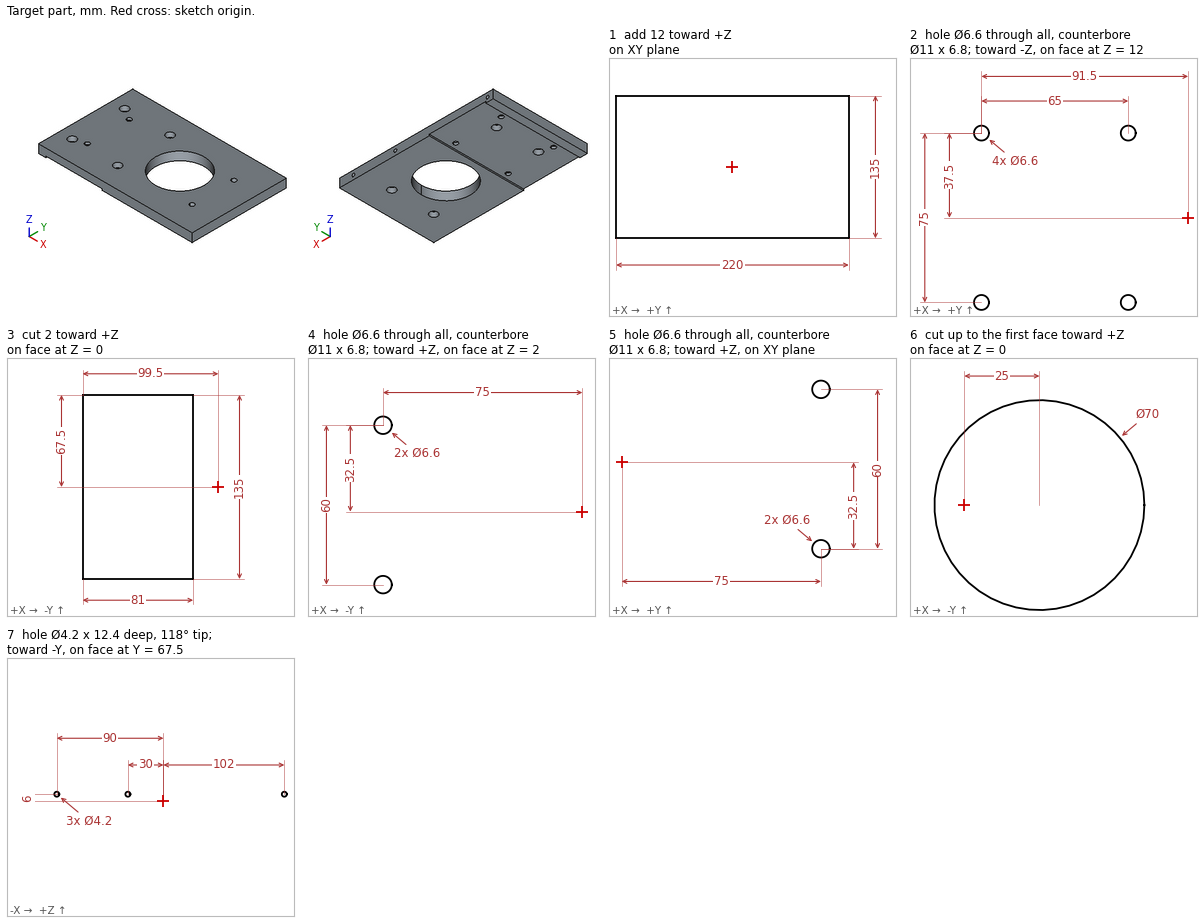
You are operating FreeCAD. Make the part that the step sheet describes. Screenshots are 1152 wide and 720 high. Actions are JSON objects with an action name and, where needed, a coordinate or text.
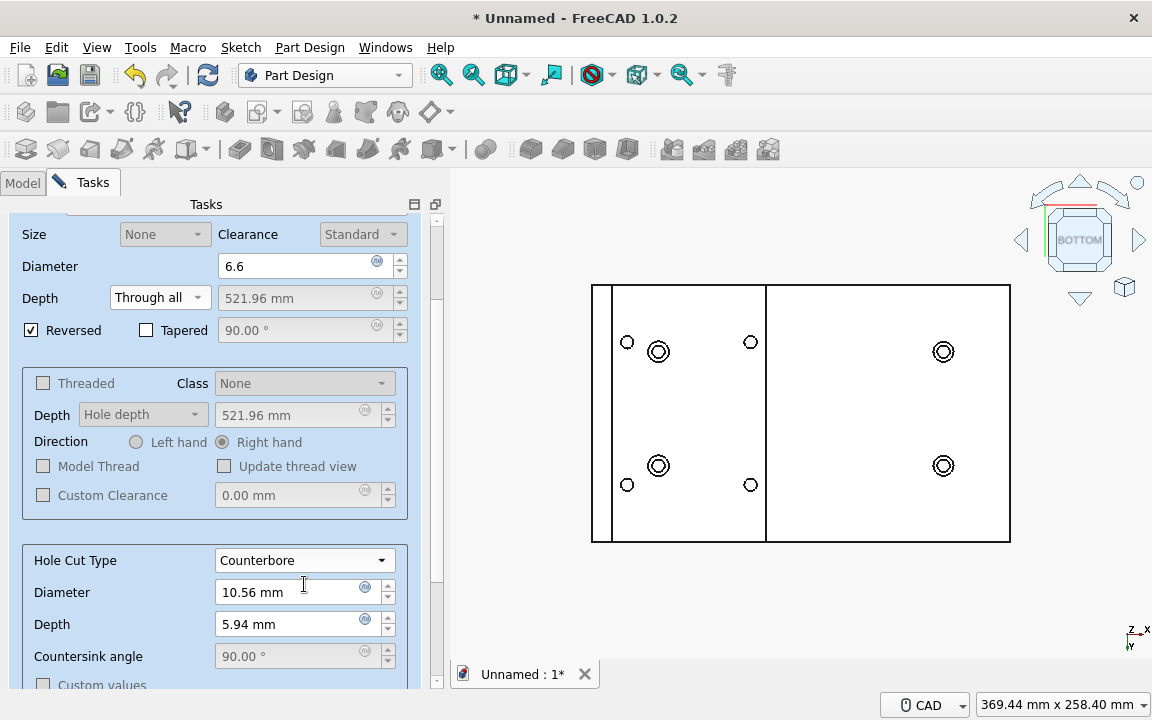
{"action": "triple_click", "coordinate": [298, 592]}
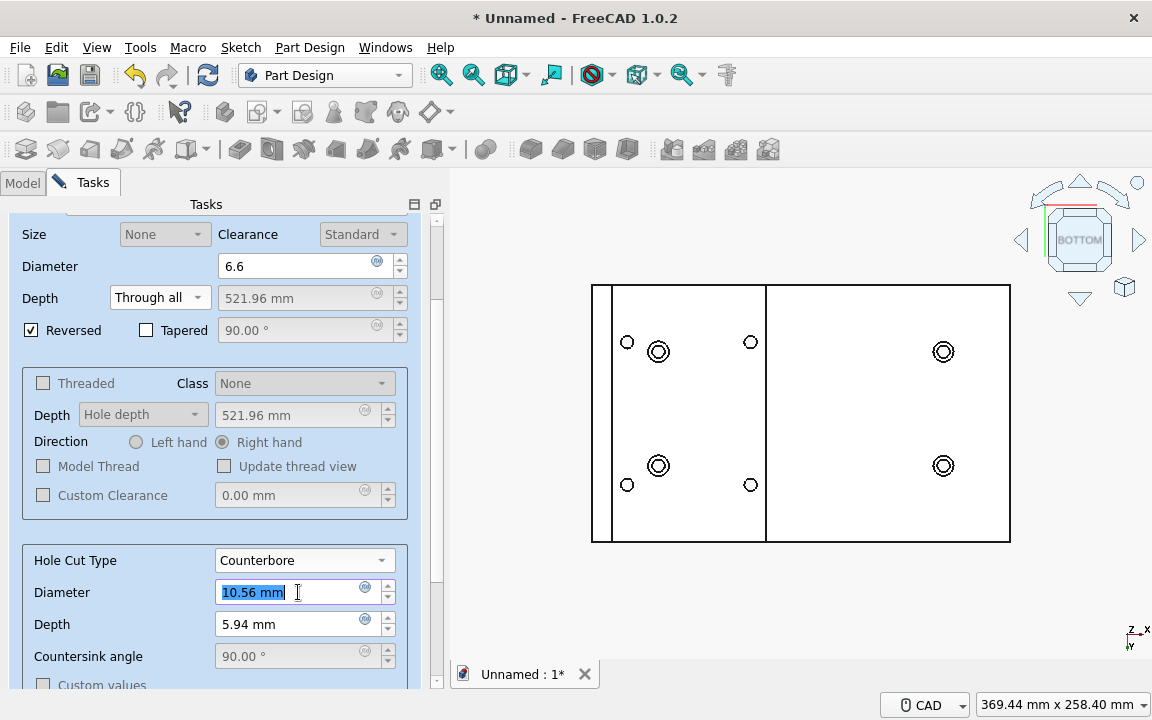
{"action": "type", "text": "11"}
{"action": "key", "text": "Tab"}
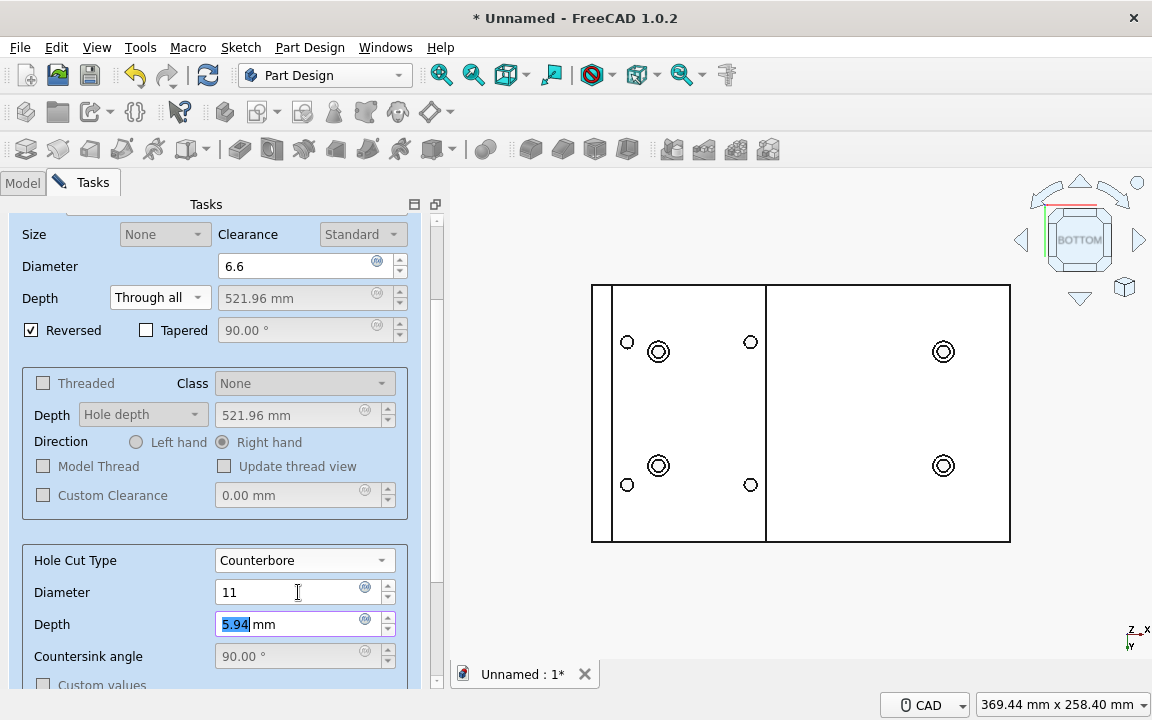
{"action": "type", "text": "6.8"}
{"action": "key", "text": "Tab"}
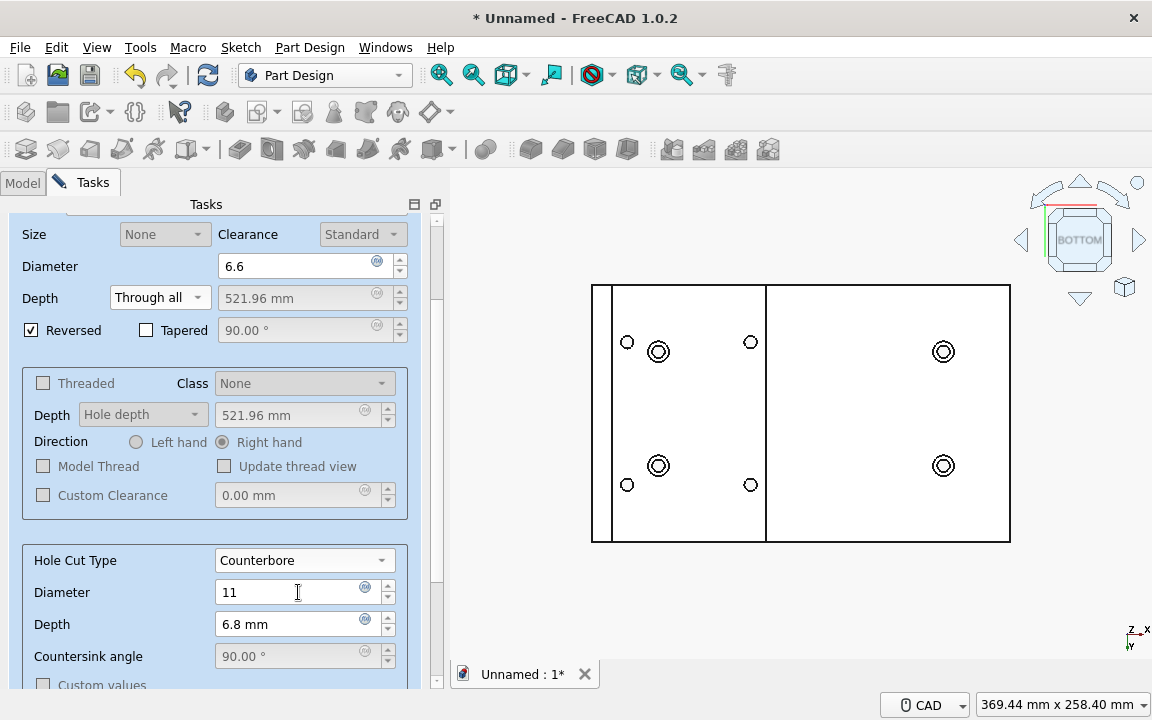
{"action": "scroll", "coordinate": [437, 451], "scroll_direction": "up", "scroll_amount": 3}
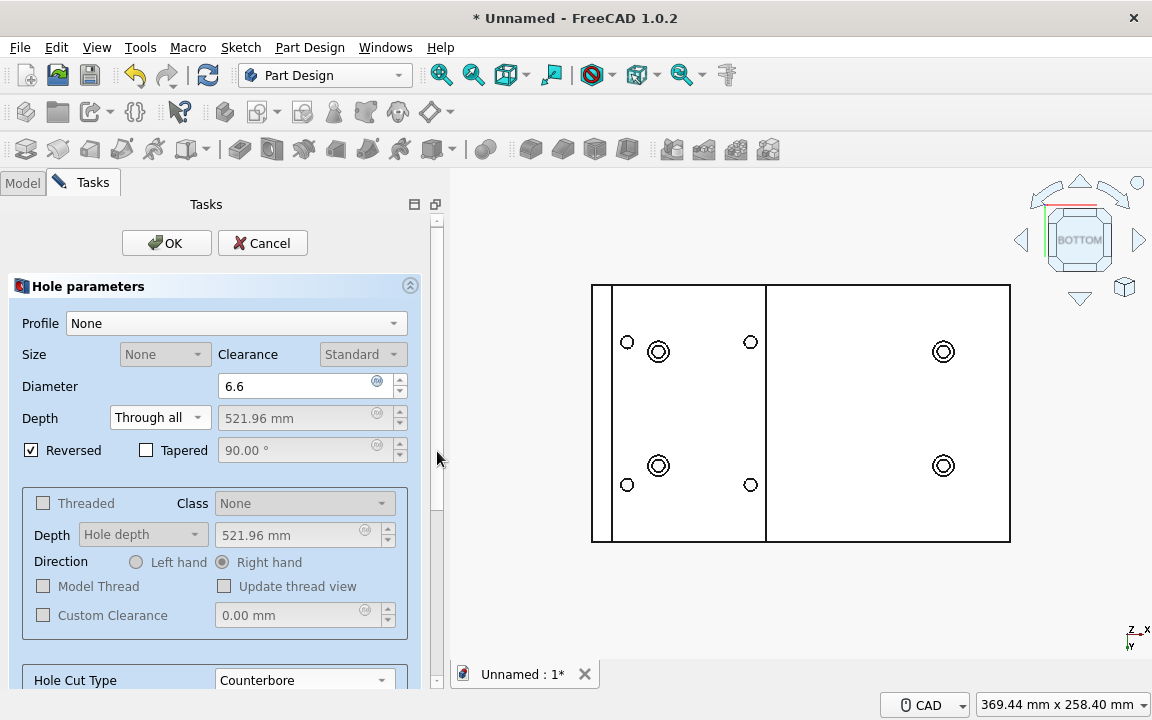
{"action": "left_click", "coordinate": [167, 243]}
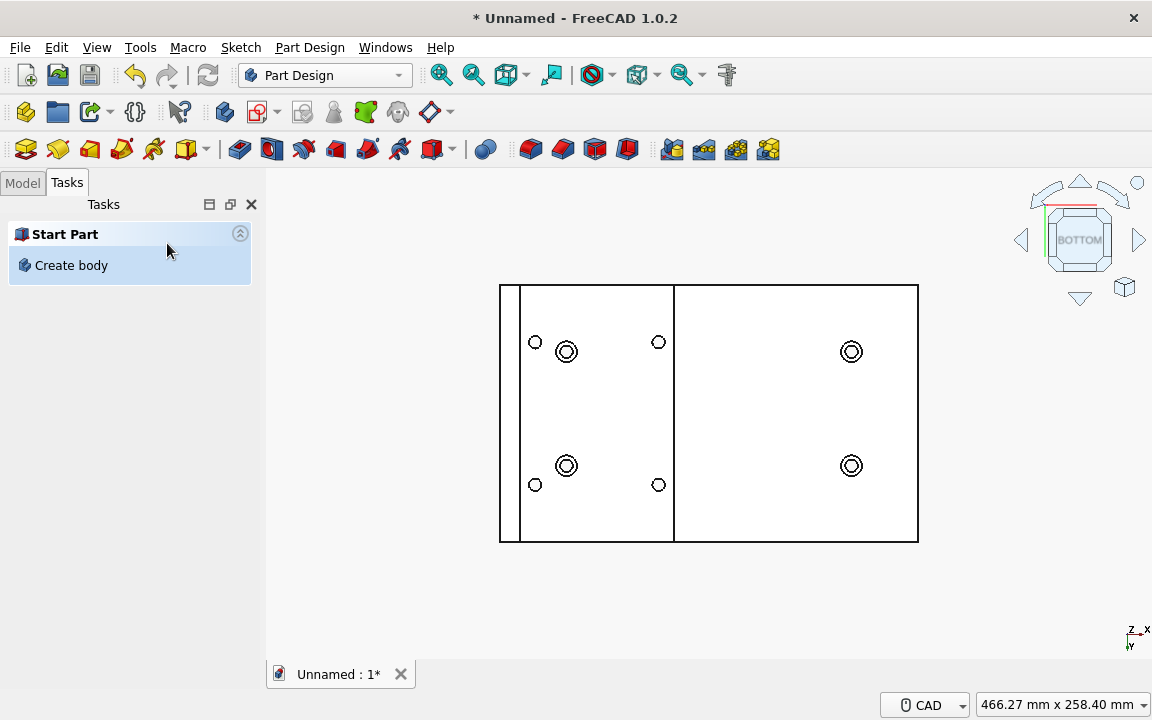
{"action": "left_click", "coordinate": [761, 413]}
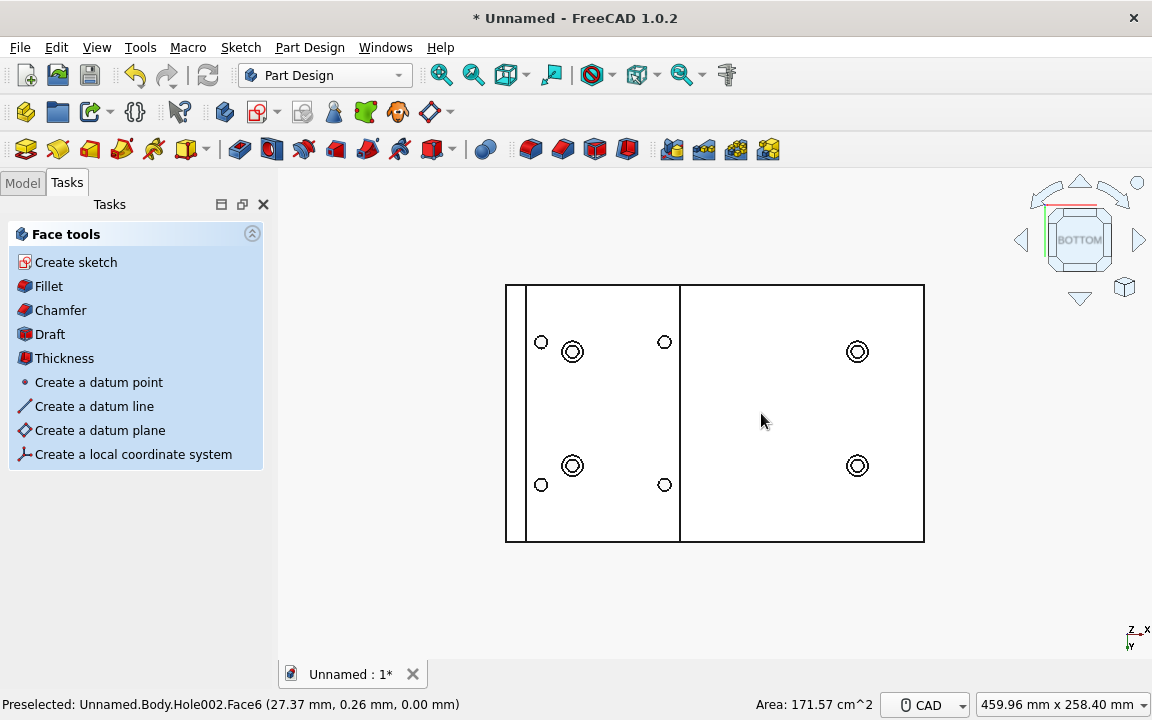
{"action": "left_click", "coordinate": [258, 112]}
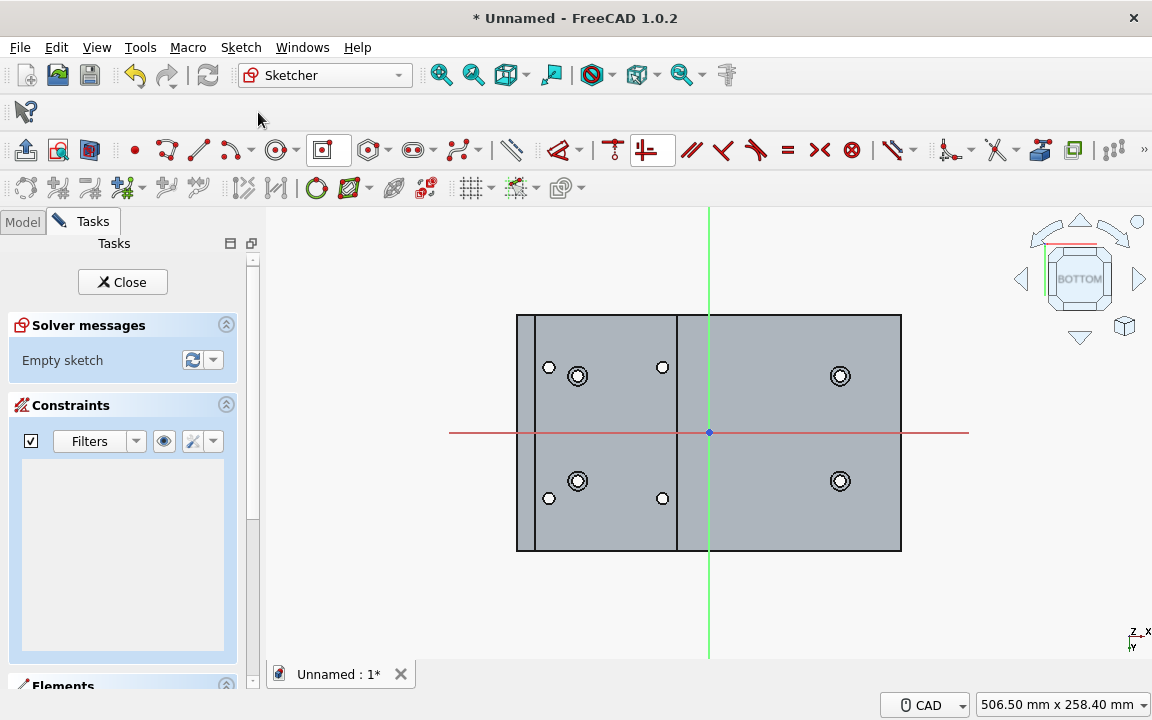
{"action": "scroll", "coordinate": [844, 433], "scroll_direction": "up", "scroll_amount": 4}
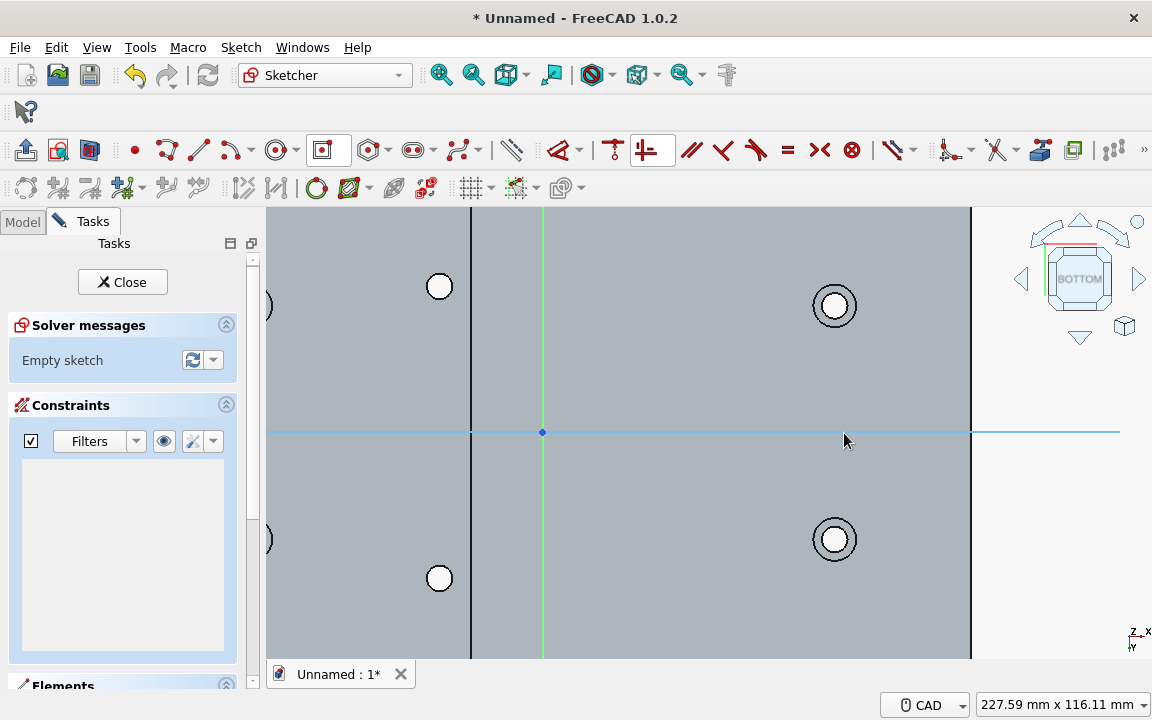
{"action": "left_click", "coordinate": [276, 150]}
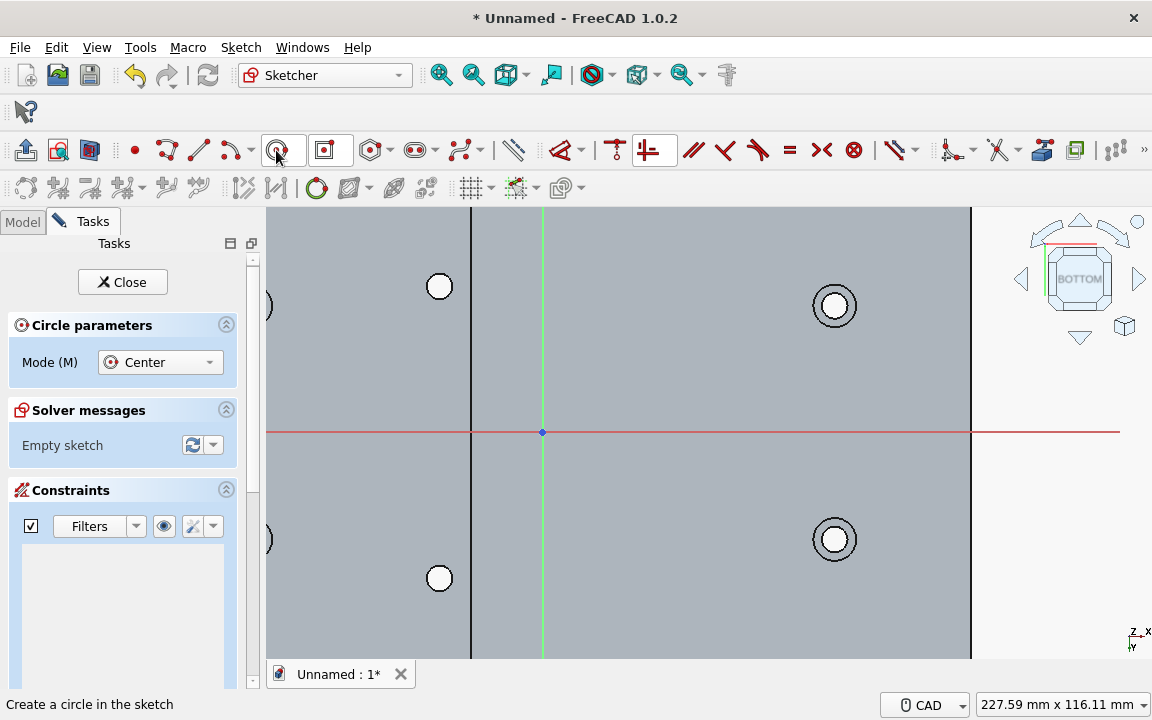
{"action": "left_click", "coordinate": [640, 432]}
{"action": "mouse_move", "coordinate": [736, 336]}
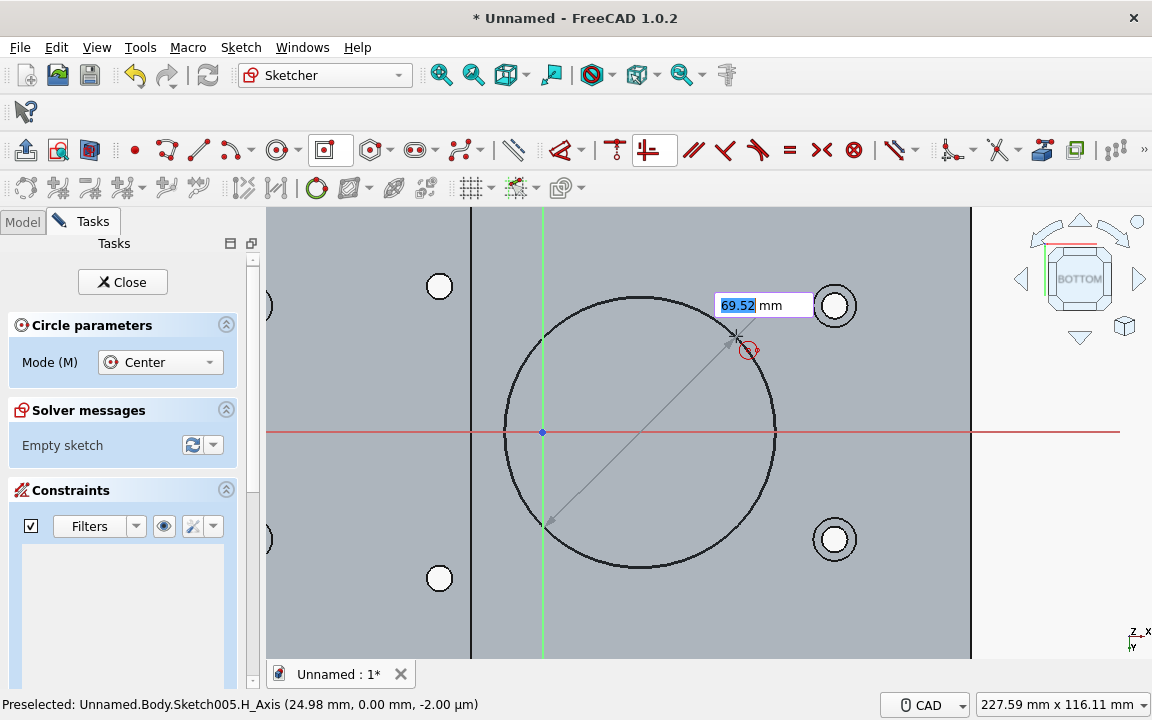
{"action": "type", "text": "70"}
{"action": "key", "text": "Return"}
{"action": "key", "text": "Escape"}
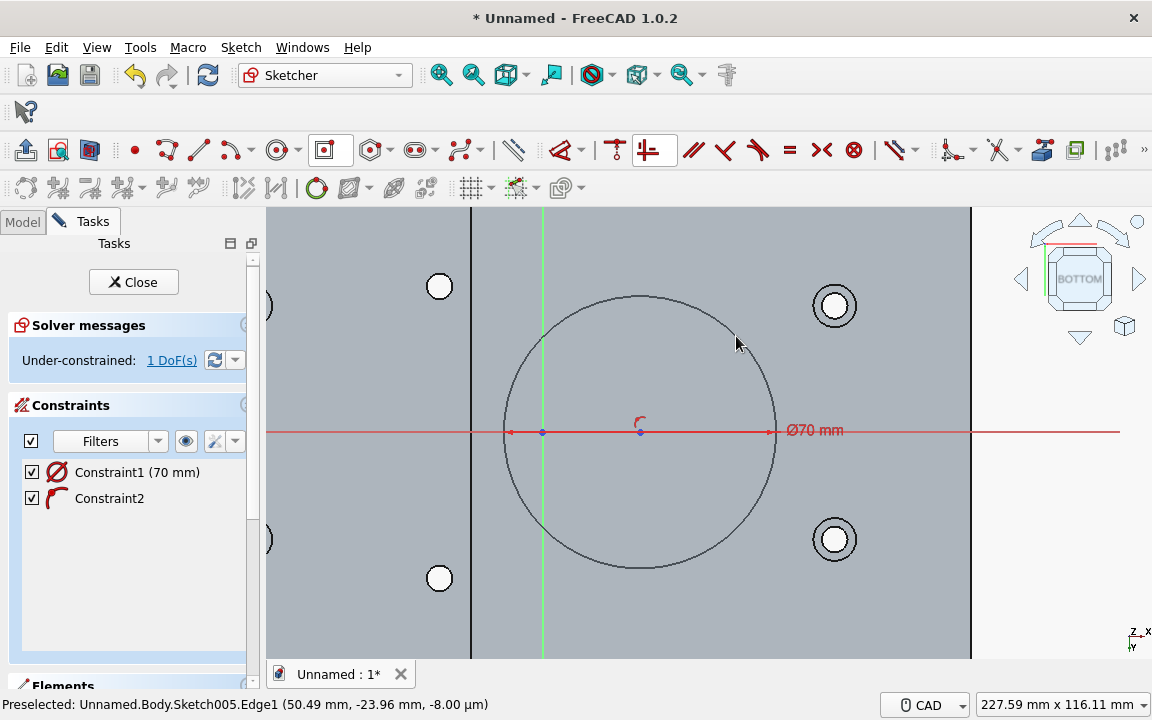
{"action": "key", "text": "d"}